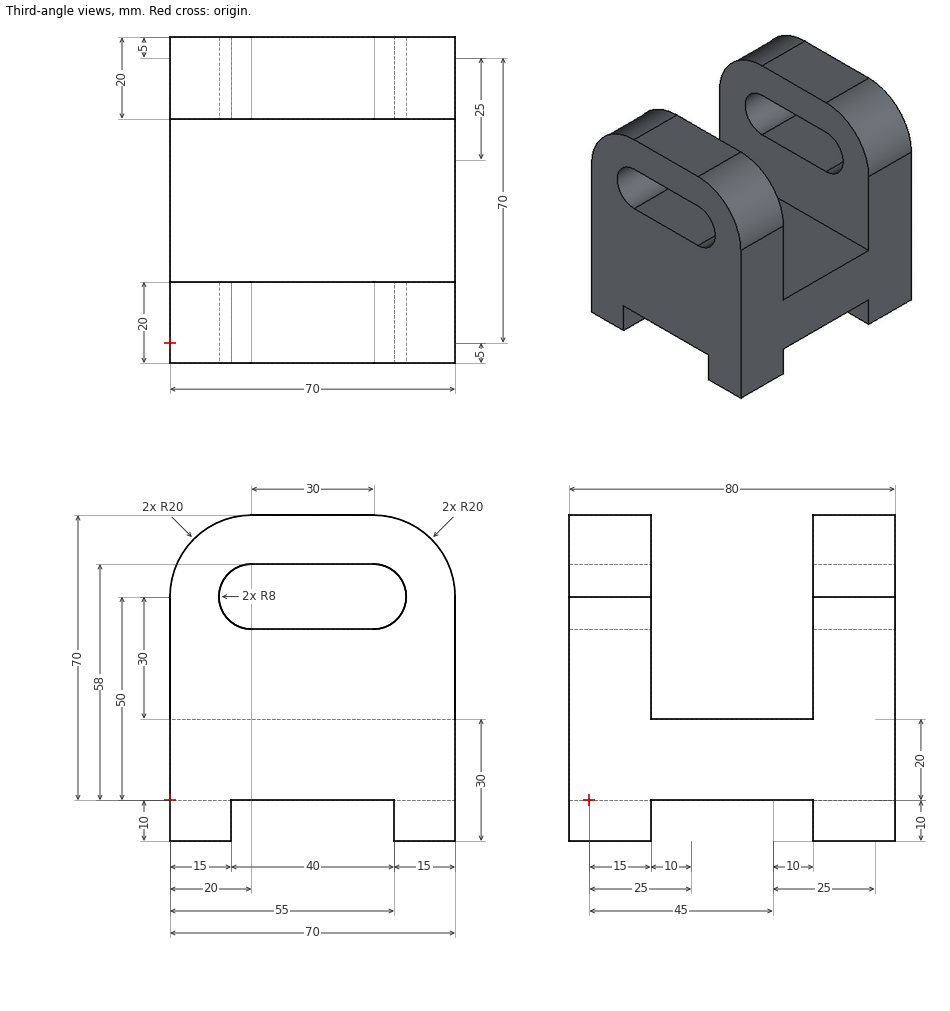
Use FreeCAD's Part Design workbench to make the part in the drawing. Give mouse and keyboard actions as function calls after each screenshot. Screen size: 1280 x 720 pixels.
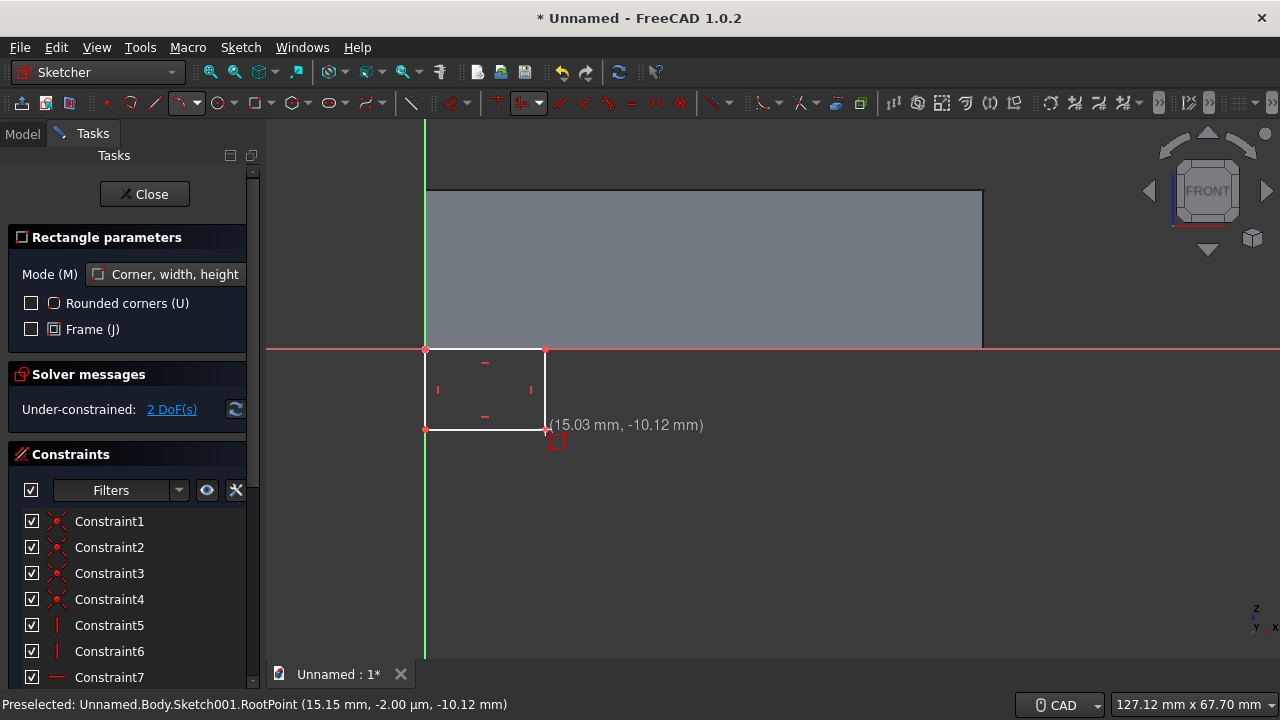
click(864, 349)
click(983, 429)
key(Escape)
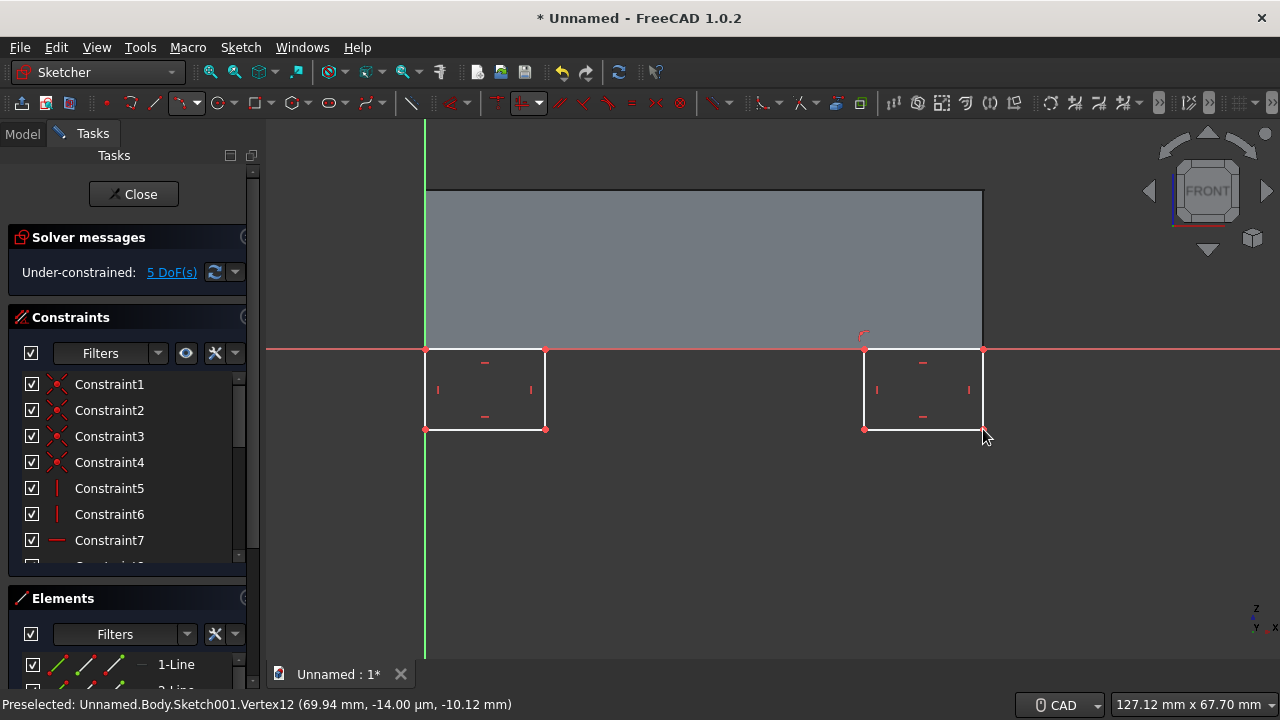
key(d)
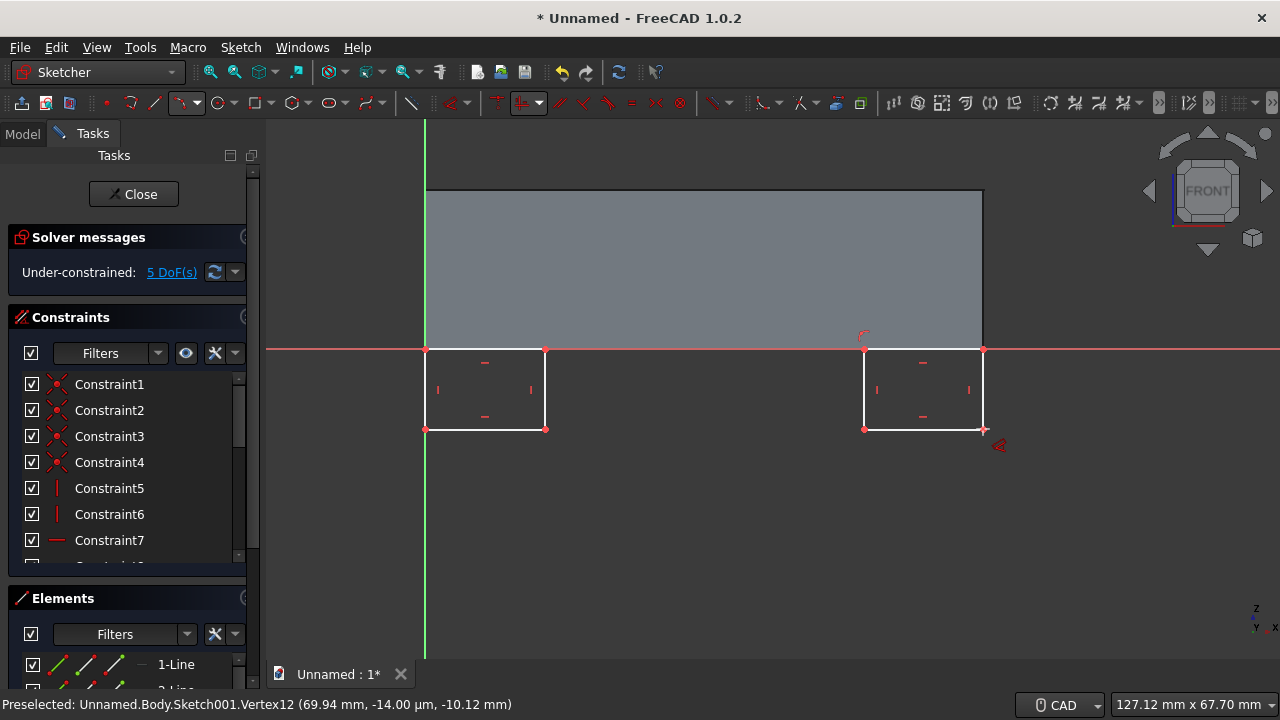
click(425, 373)
click(391, 390)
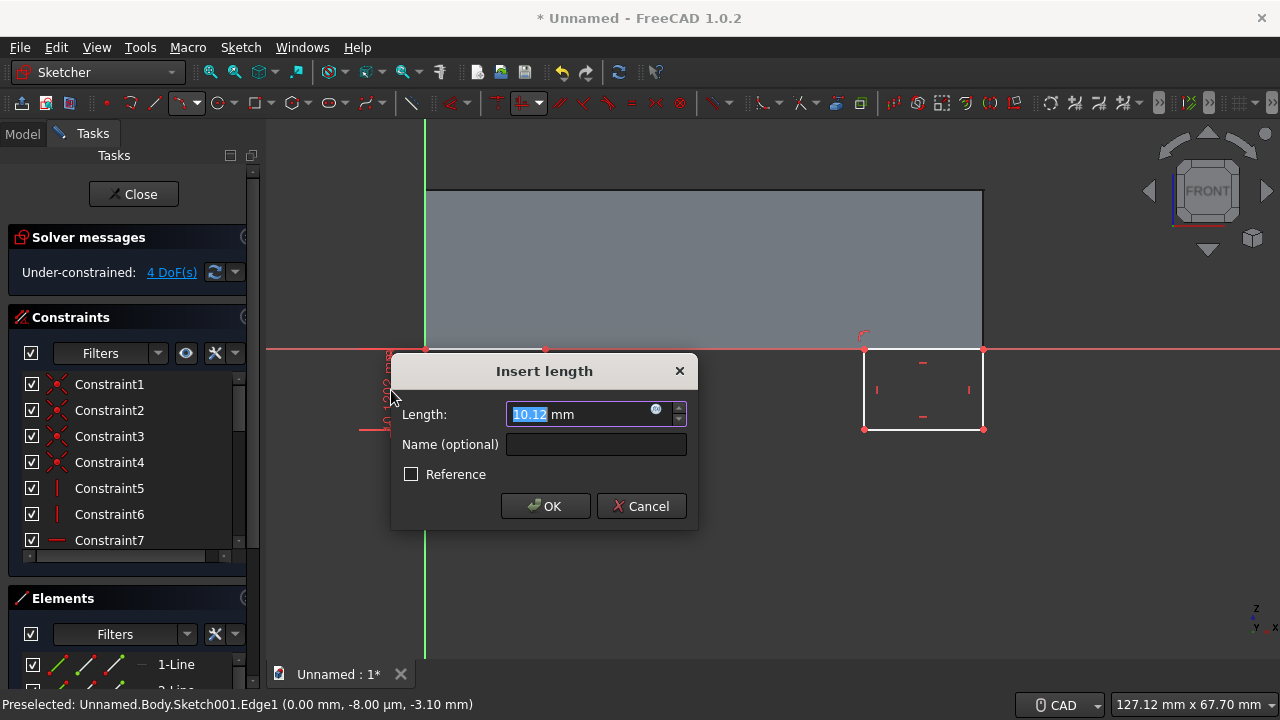
text(10)
key(Return)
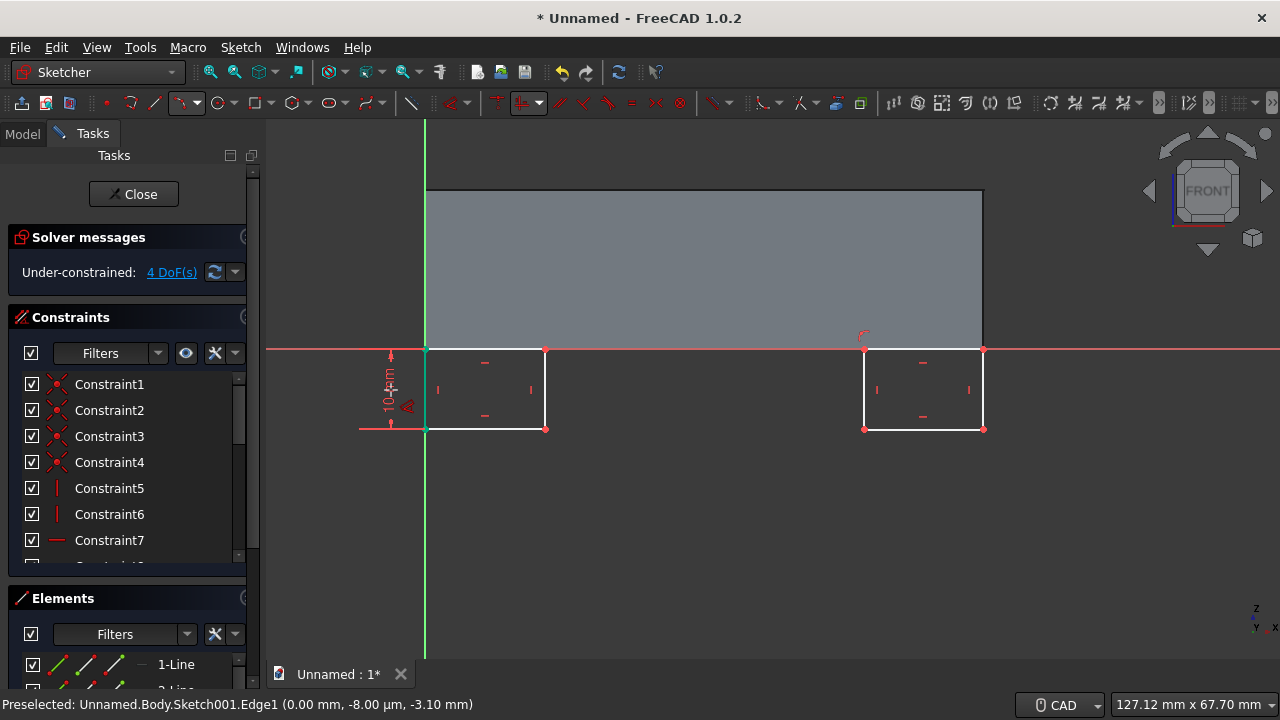
click(461, 429)
click(485, 463)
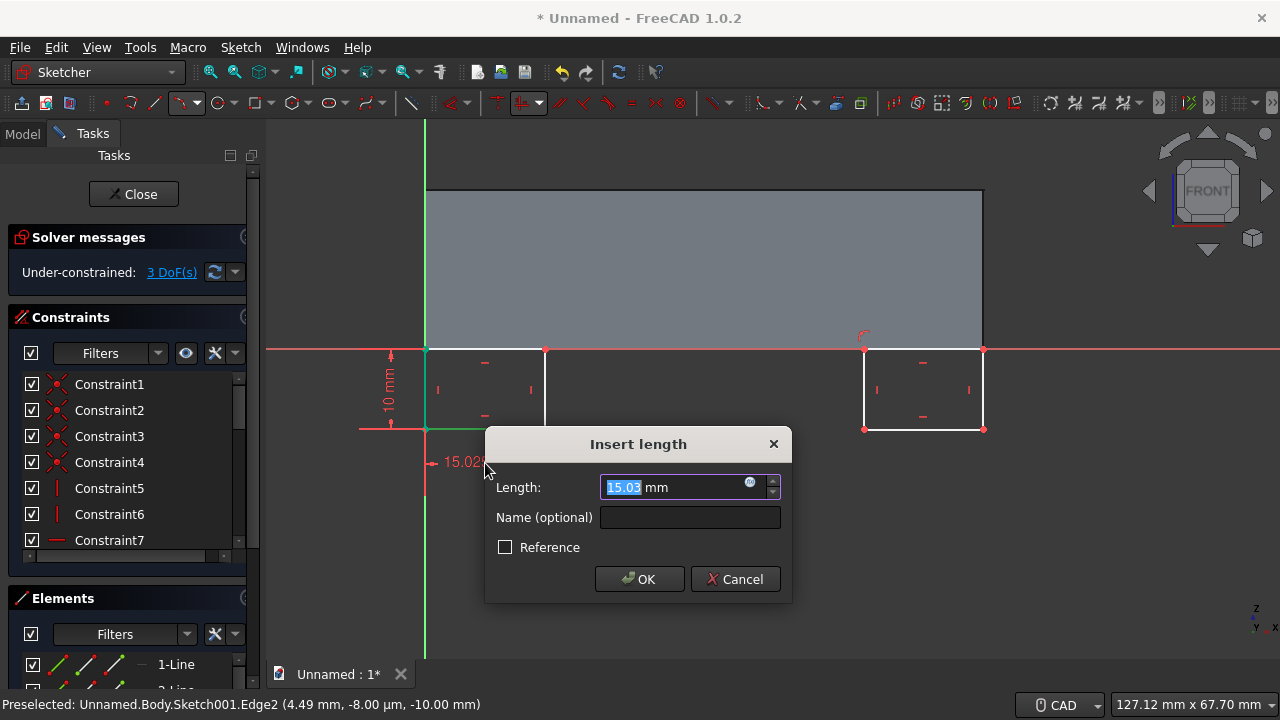
text(15)
key(Return)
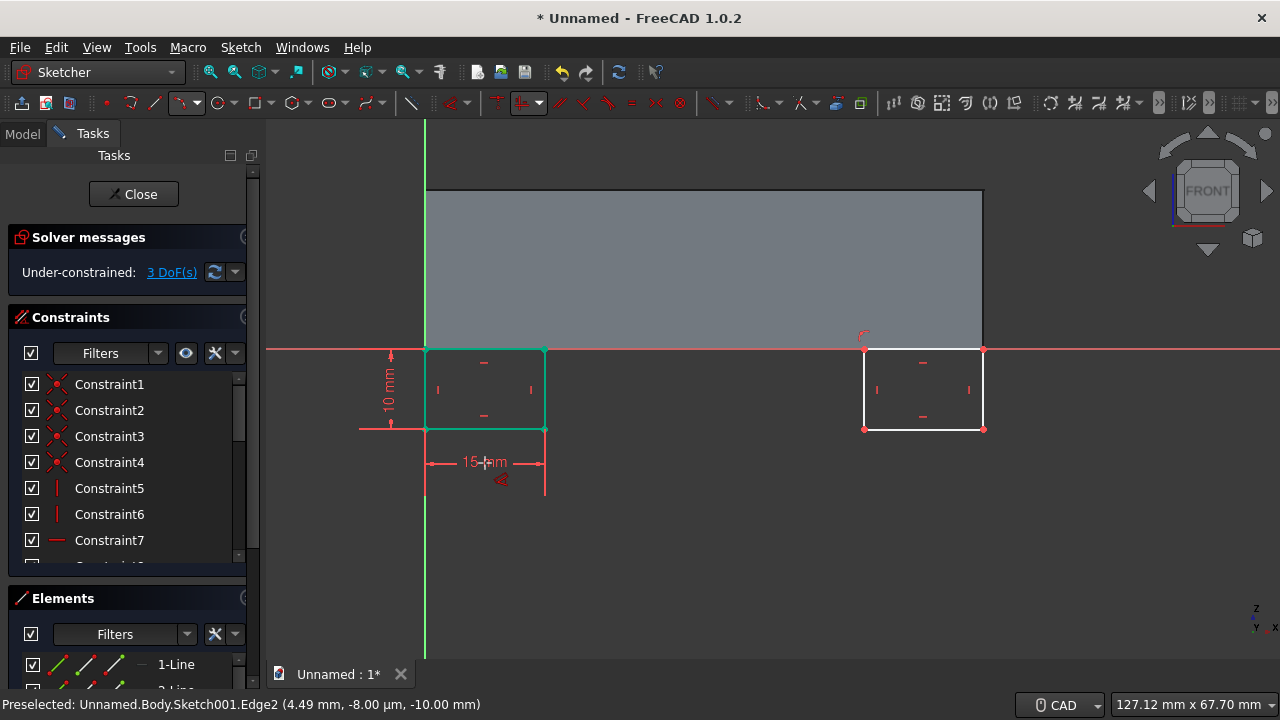
click(864, 373)
click(898, 390)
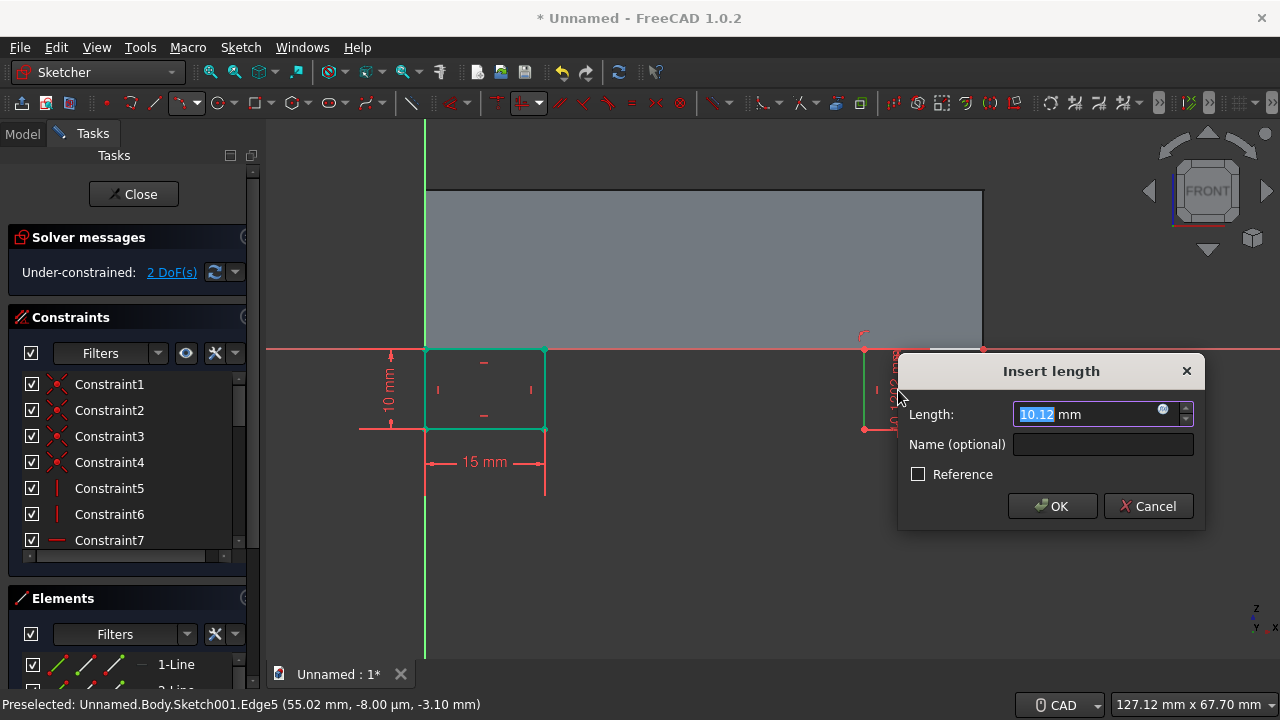
text(10)
key(Return)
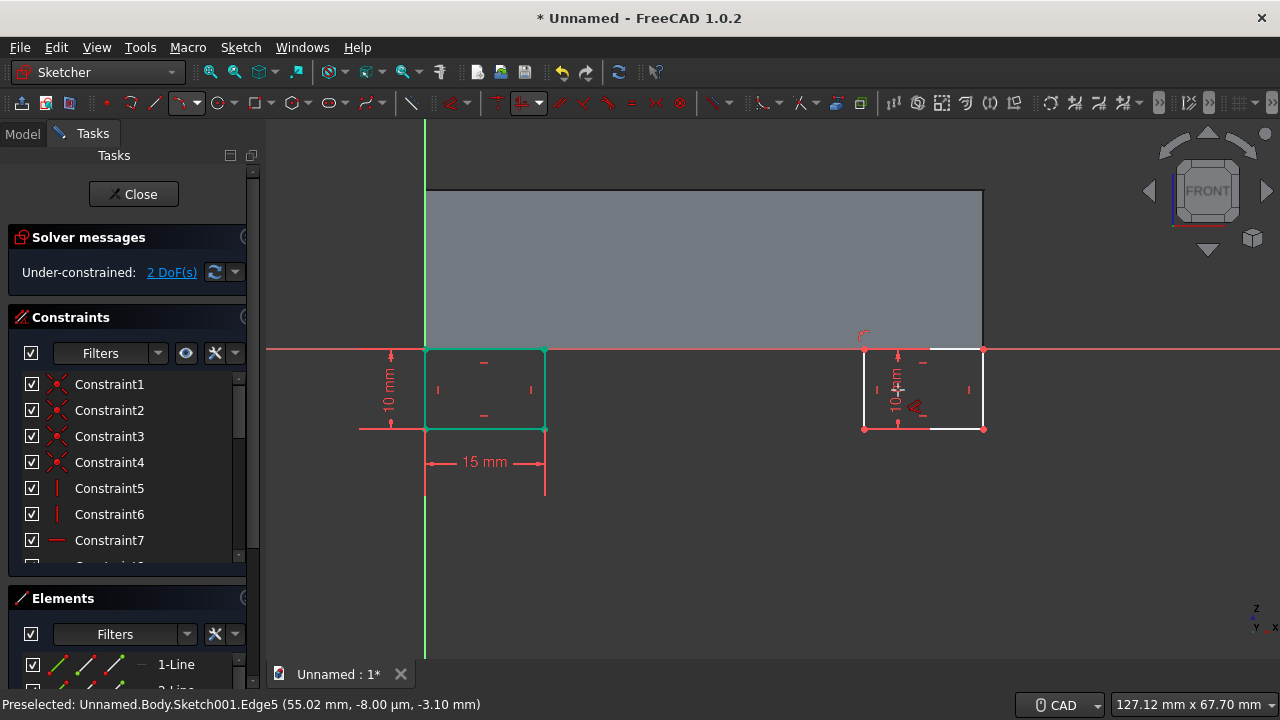
click(900, 429)
click(923, 463)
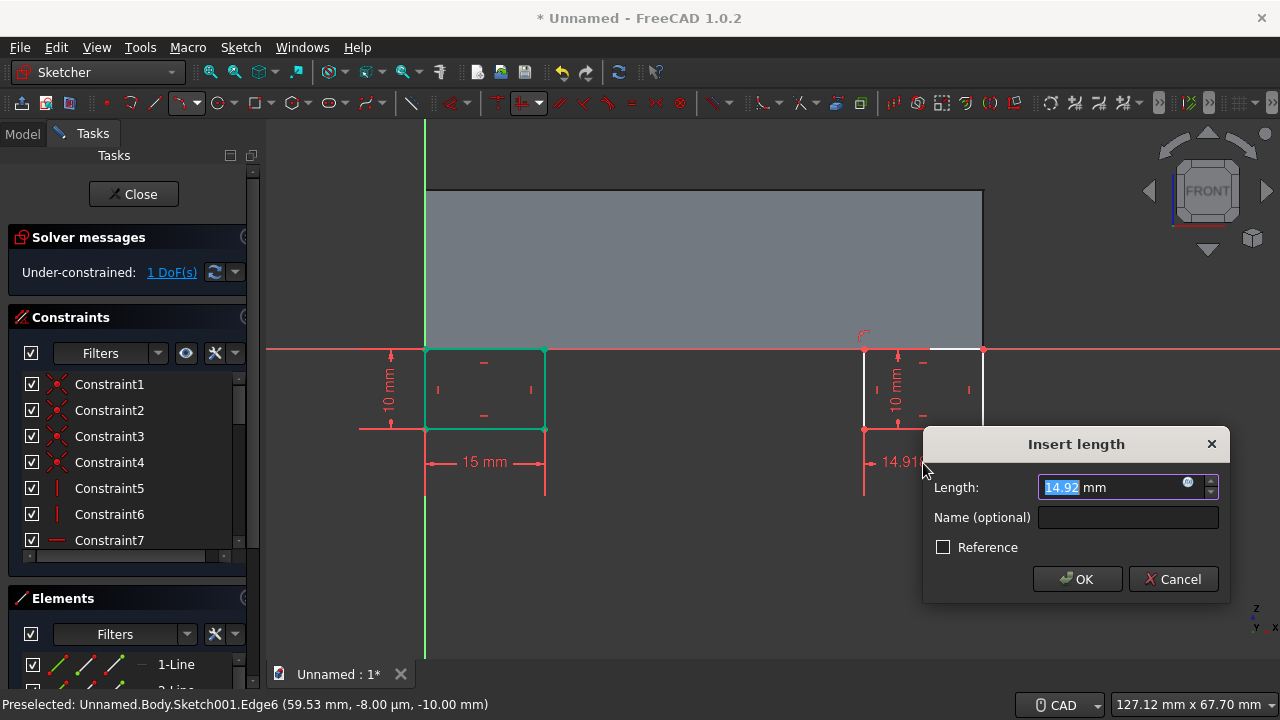
text(15)
key(Return)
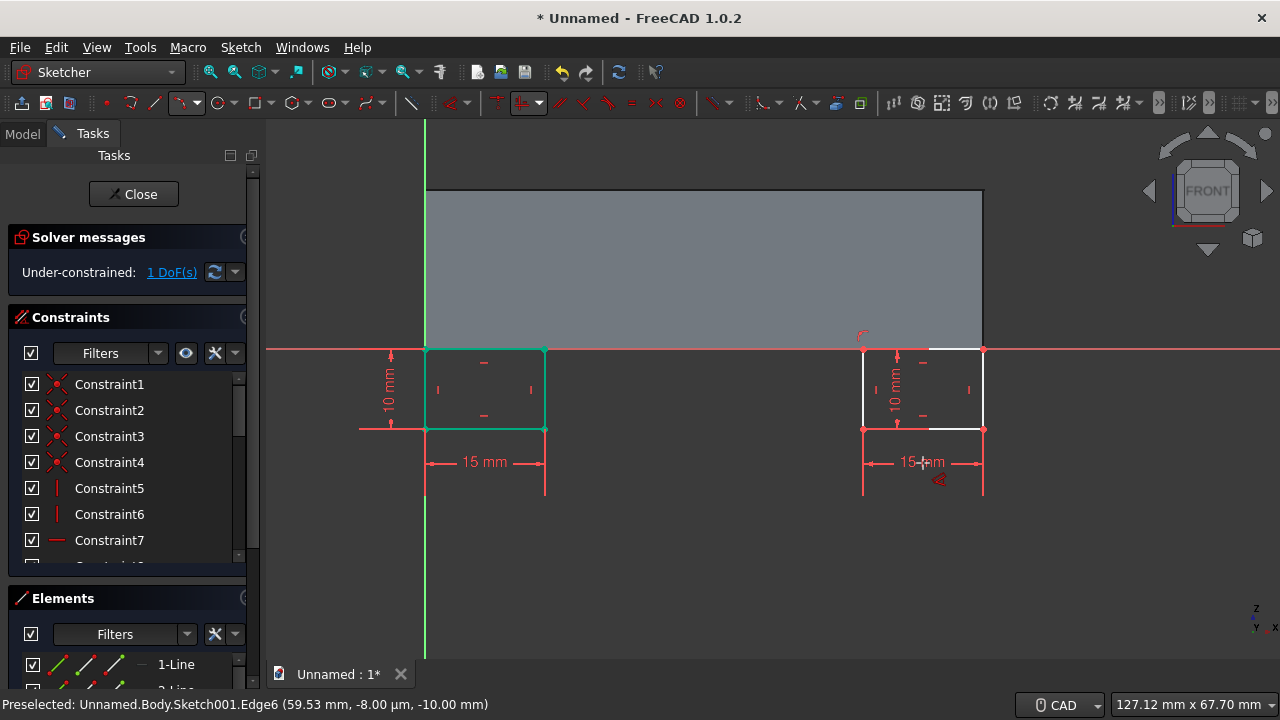
click(863, 349)
click(644, 315)